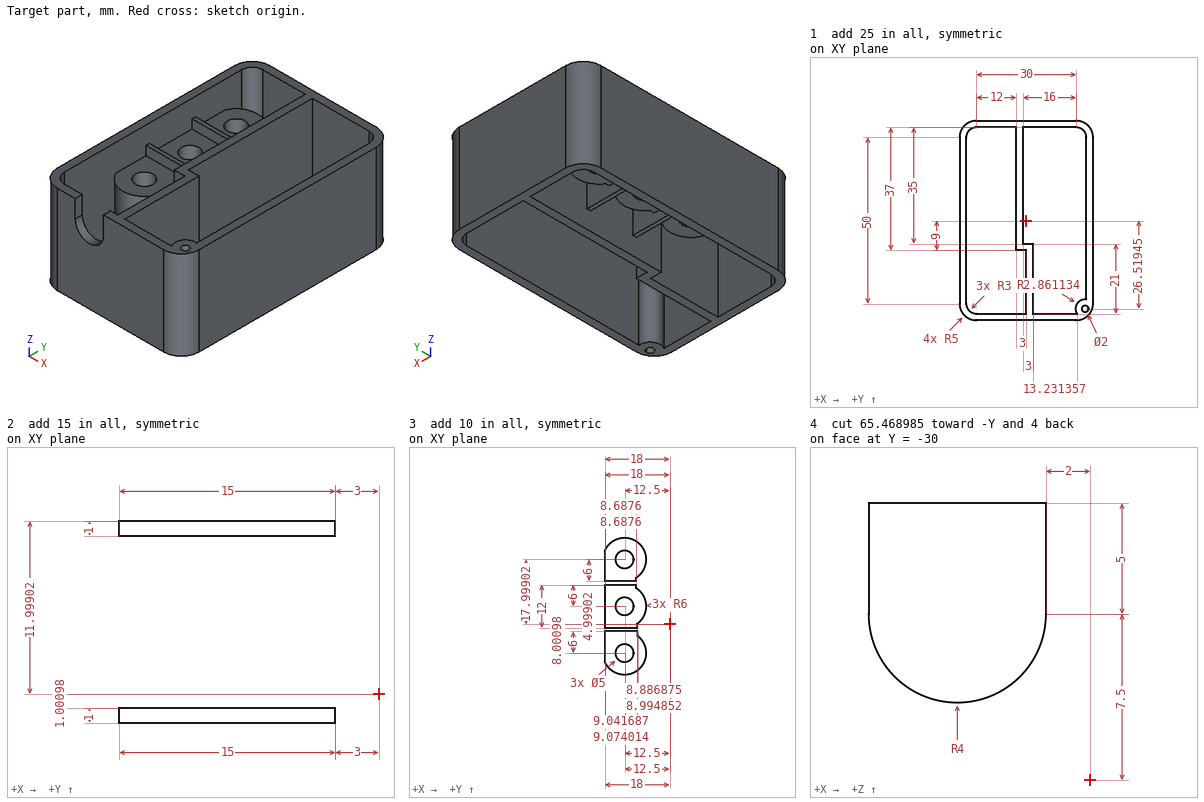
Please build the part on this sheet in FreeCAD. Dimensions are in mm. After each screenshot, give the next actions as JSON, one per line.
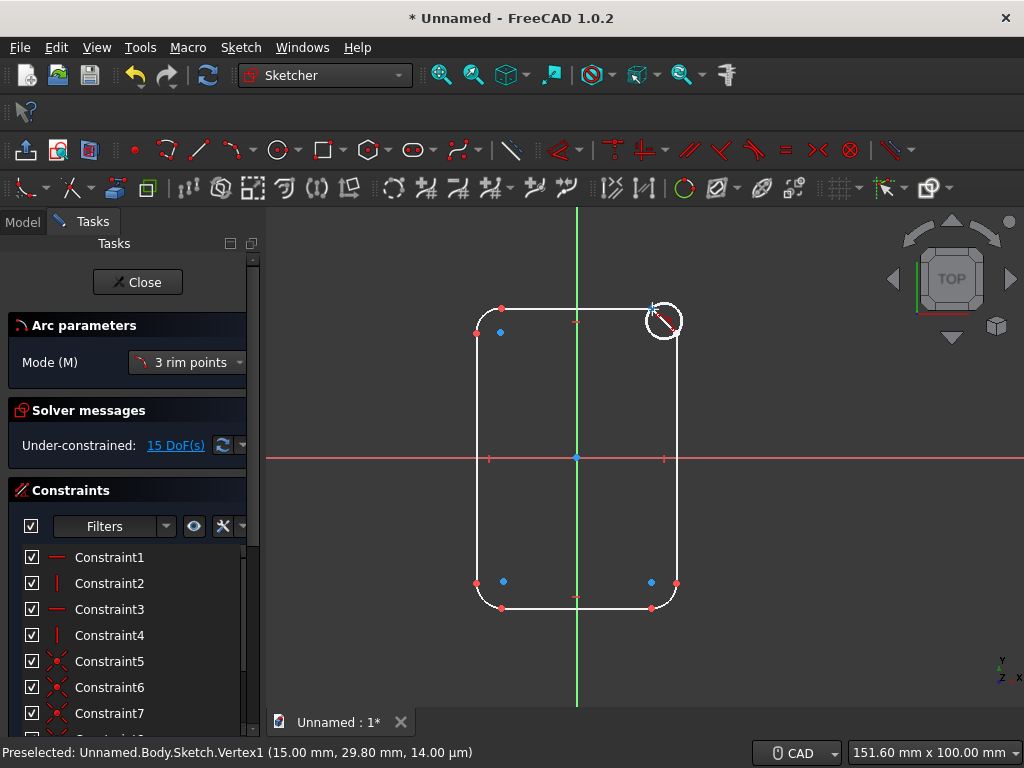
{"action": "scroll", "coordinate": [669, 315], "scroll_direction": "up", "scroll_amount": 4}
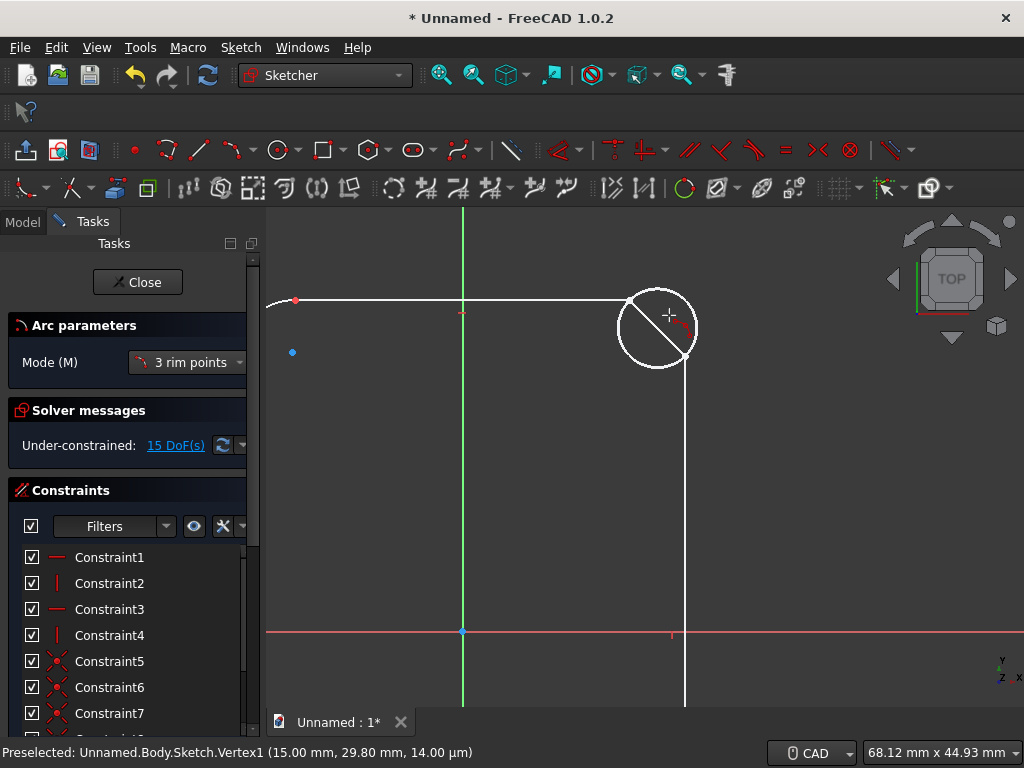
{"action": "left_click", "coordinate": [669, 314]}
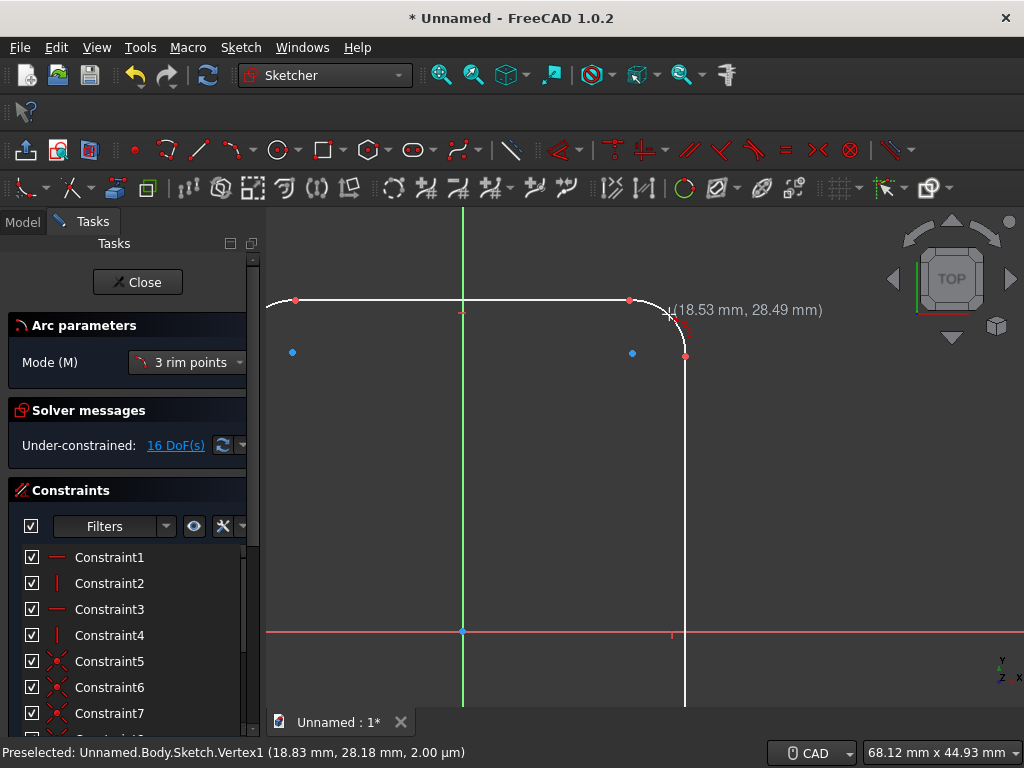
{"action": "left_click", "coordinate": [200, 150]}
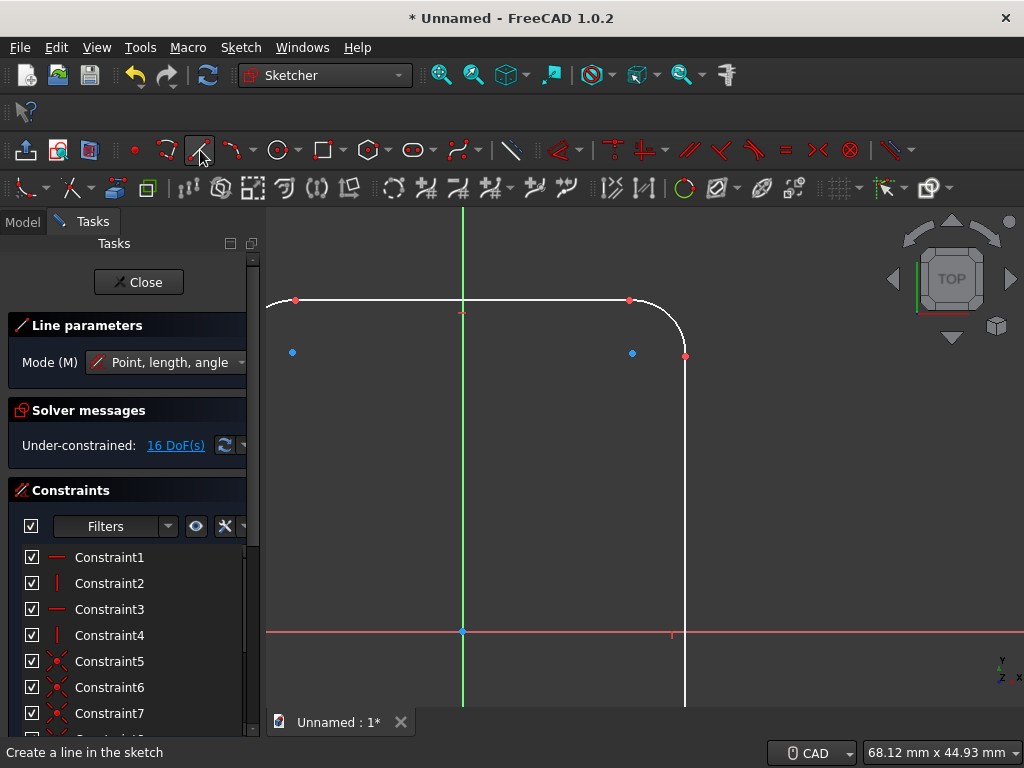
{"action": "scroll", "coordinate": [669, 314], "scroll_direction": "down", "scroll_amount": 4}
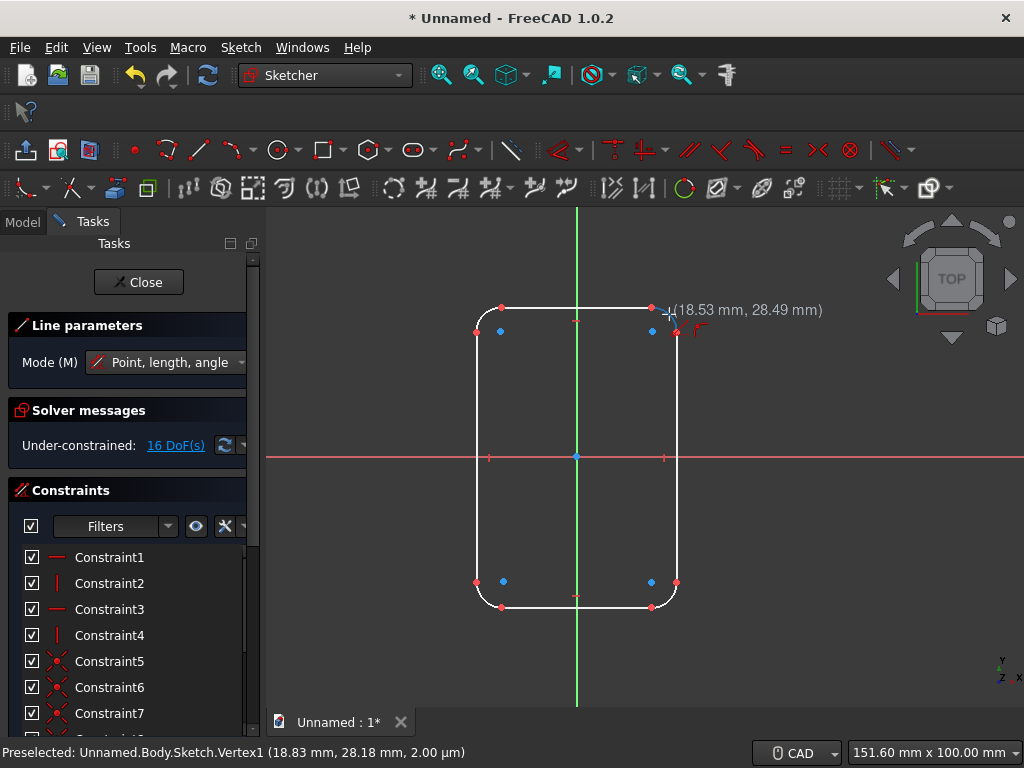
{"action": "scroll", "coordinate": [487, 582], "scroll_direction": "up", "scroll_amount": 3}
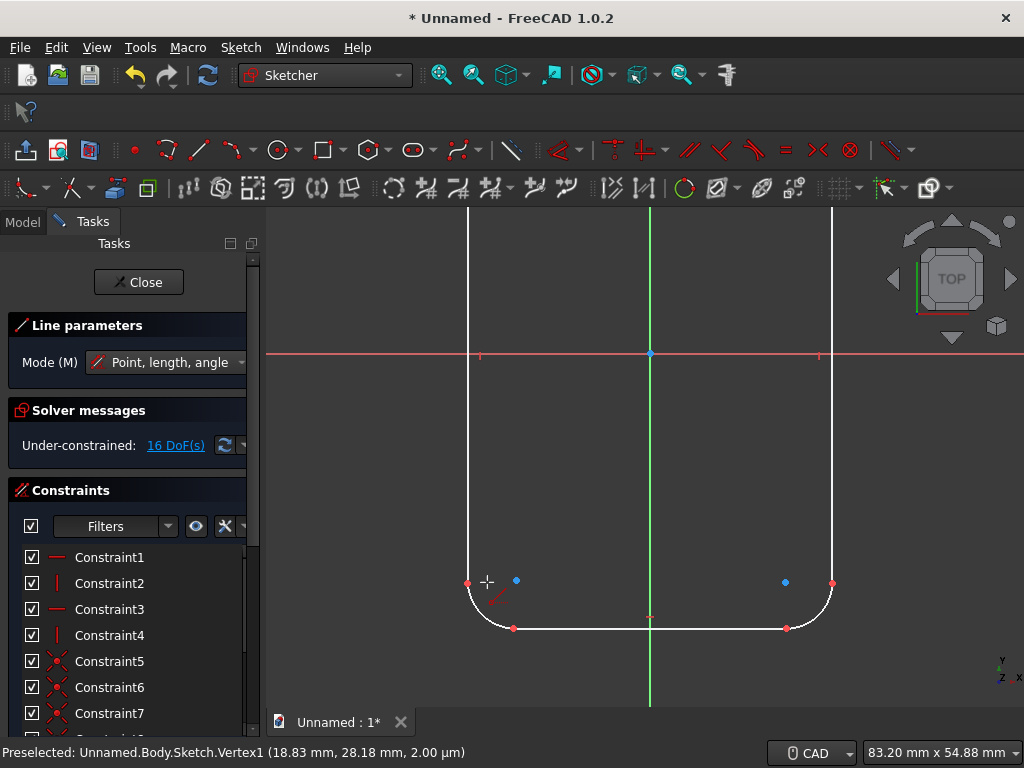
{"action": "left_click", "coordinate": [486, 581]}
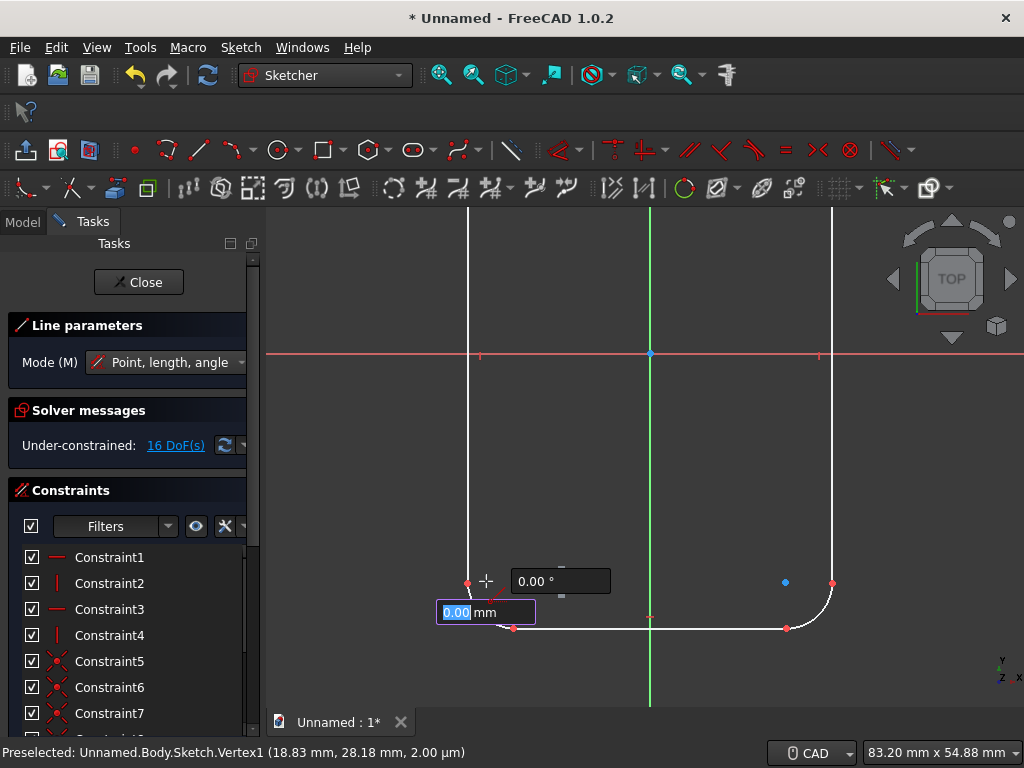
{"action": "scroll", "coordinate": [487, 583], "scroll_direction": "down", "scroll_amount": 3}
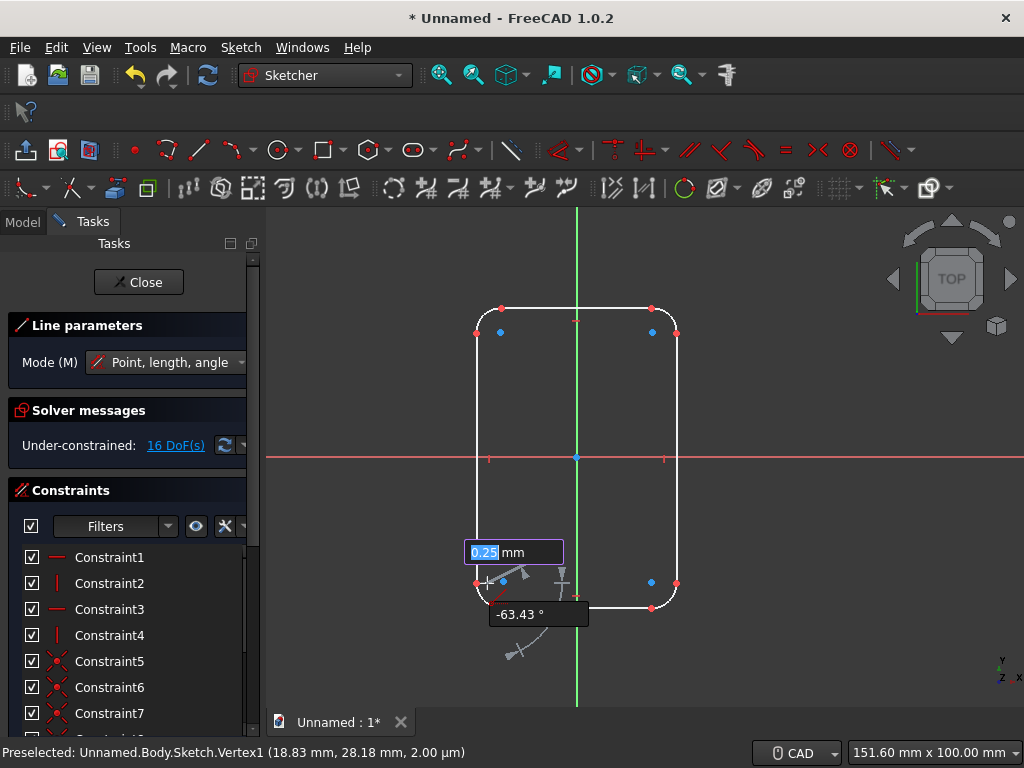
{"action": "scroll", "coordinate": [487, 332], "scroll_direction": "up", "scroll_amount": 3}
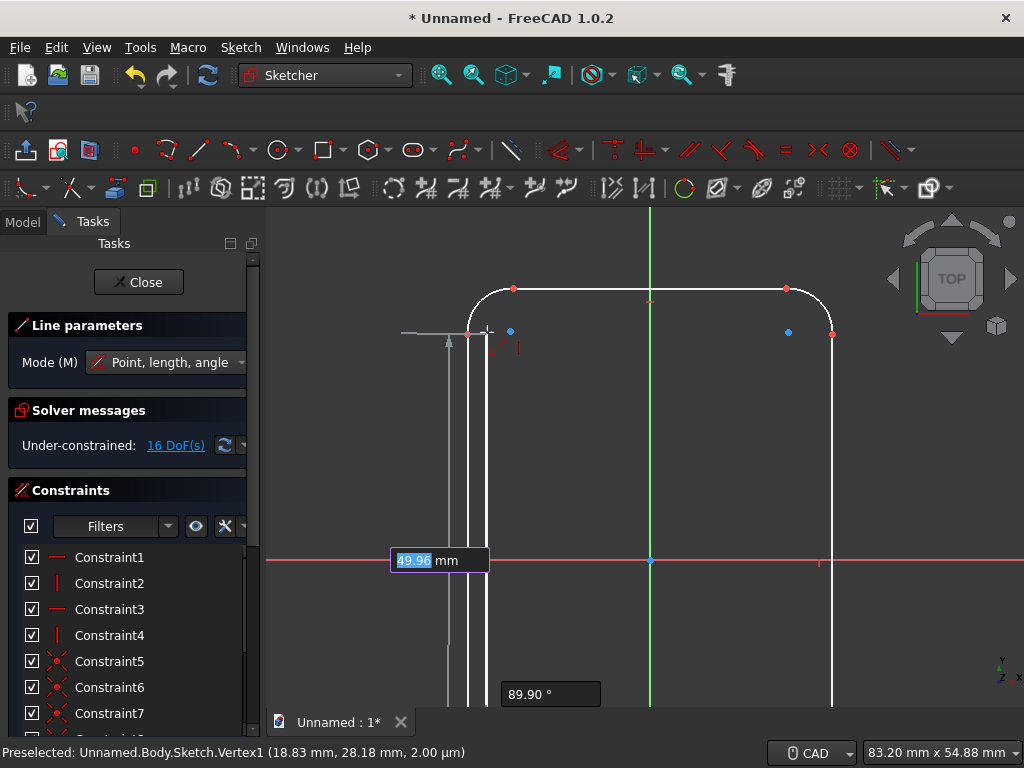
{"action": "left_click", "coordinate": [486, 333]}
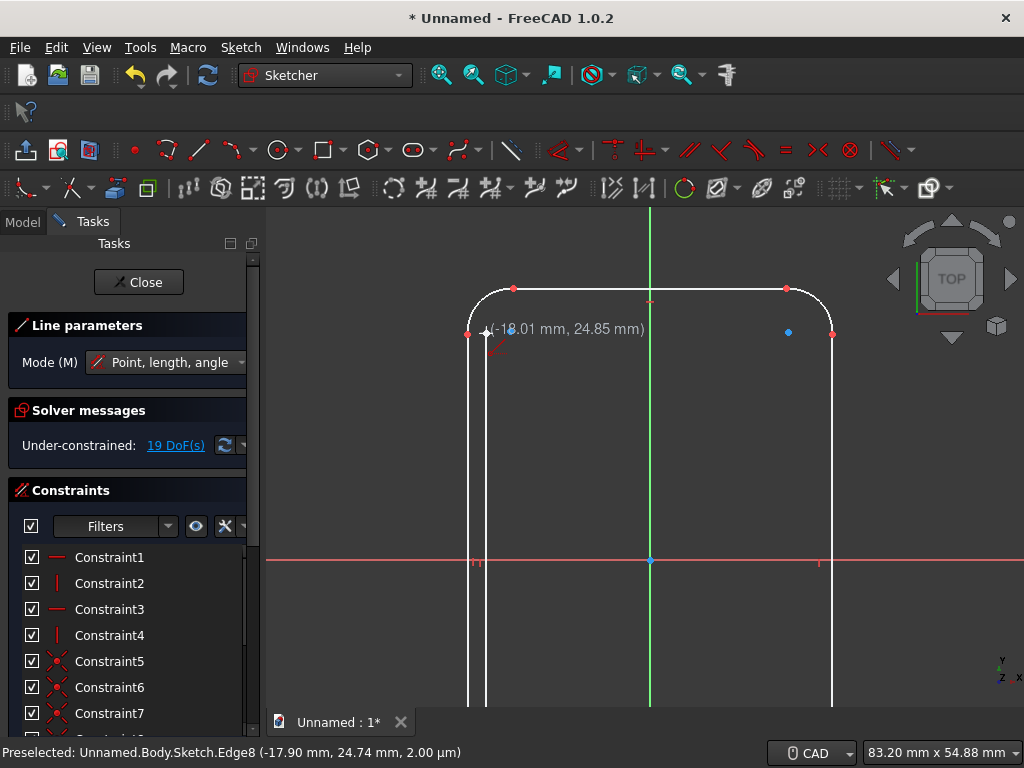
{"action": "left_click", "coordinate": [168, 150]}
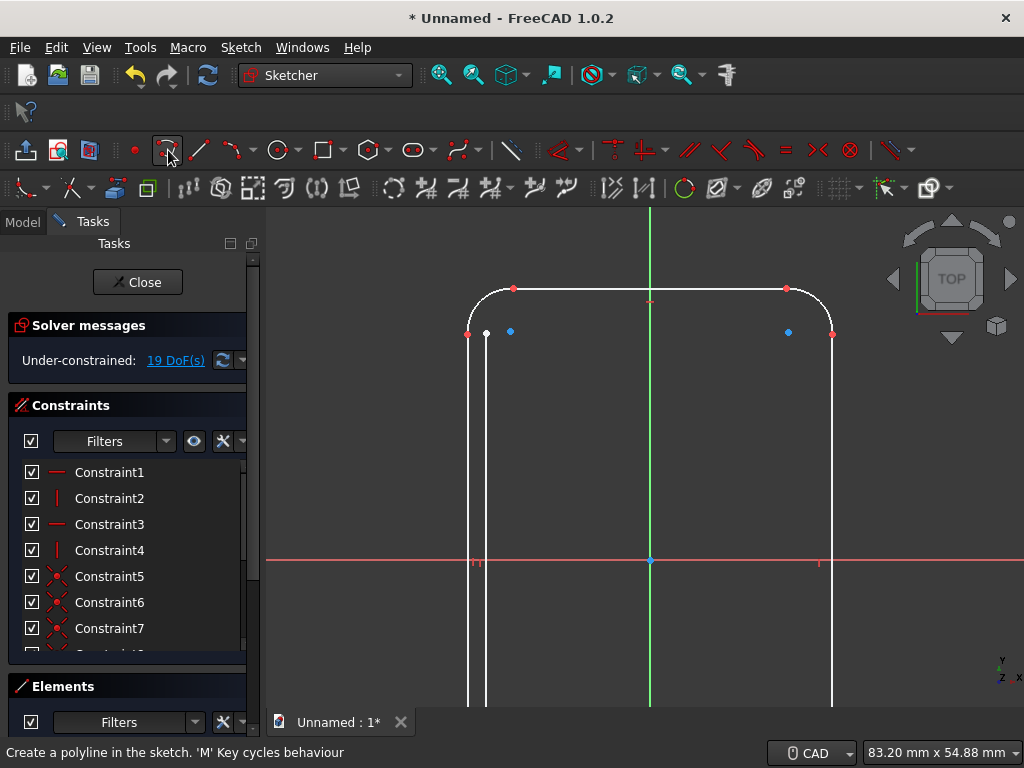
{"action": "left_click", "coordinate": [513, 305]}
{"action": "left_click", "coordinate": [623, 305]}
{"action": "left_click", "coordinate": [623, 642]}
{"action": "left_click", "coordinate": [650, 642]}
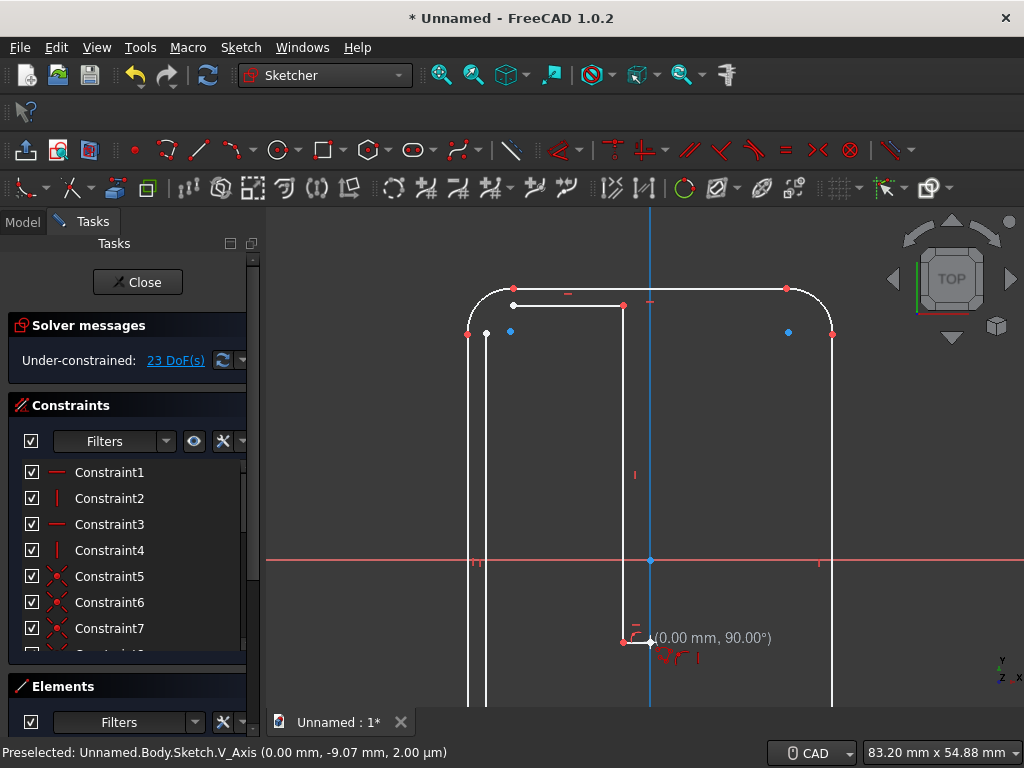
{"action": "scroll", "coordinate": [487, 331], "scroll_direction": "down", "scroll_amount": 3}